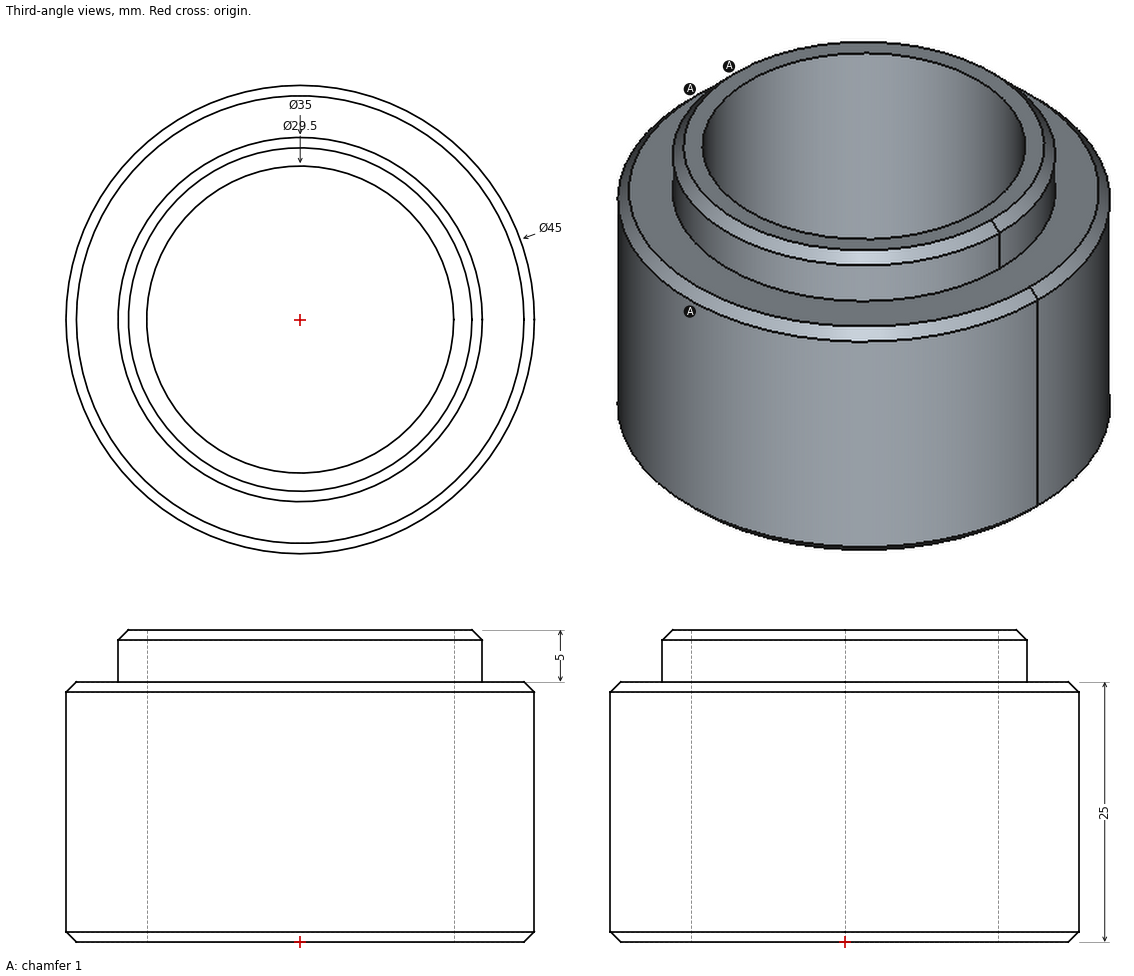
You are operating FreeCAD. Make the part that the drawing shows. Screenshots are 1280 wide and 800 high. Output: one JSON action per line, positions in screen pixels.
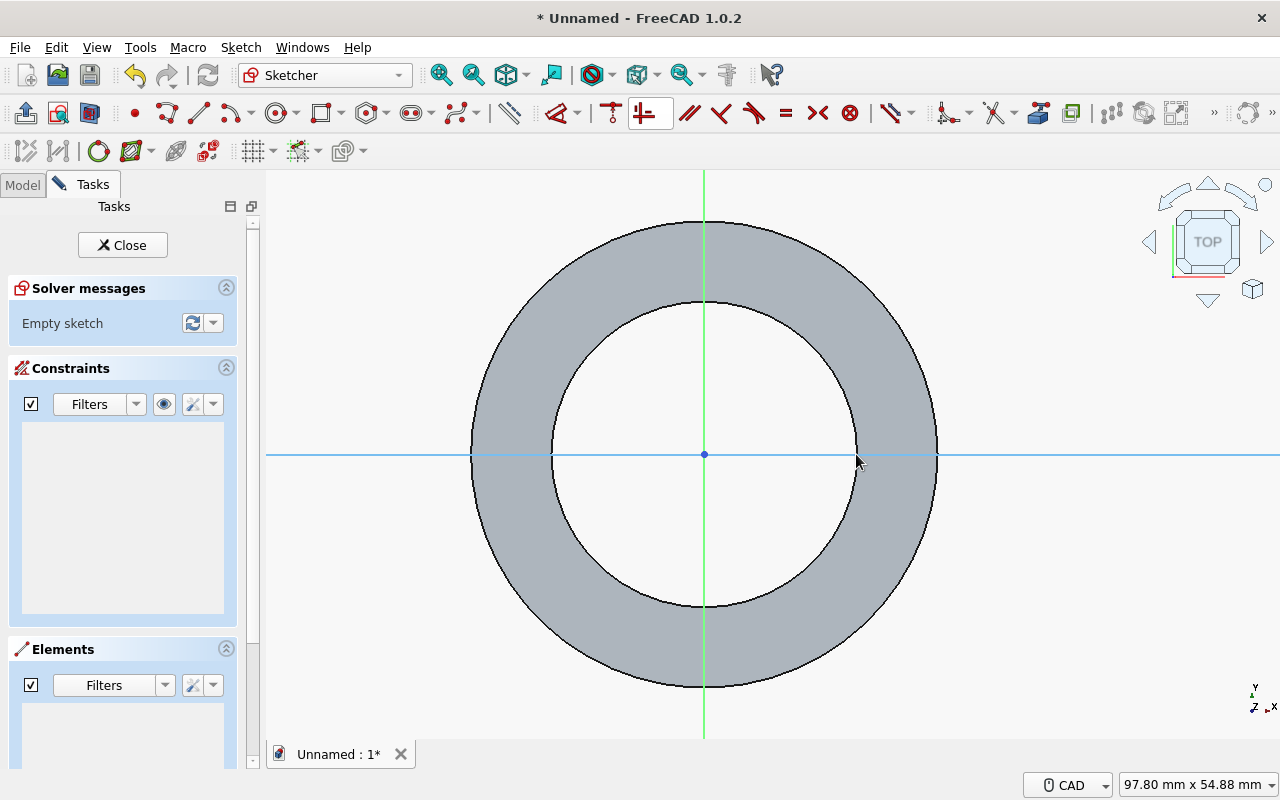
{"action": "key", "text": "g c"}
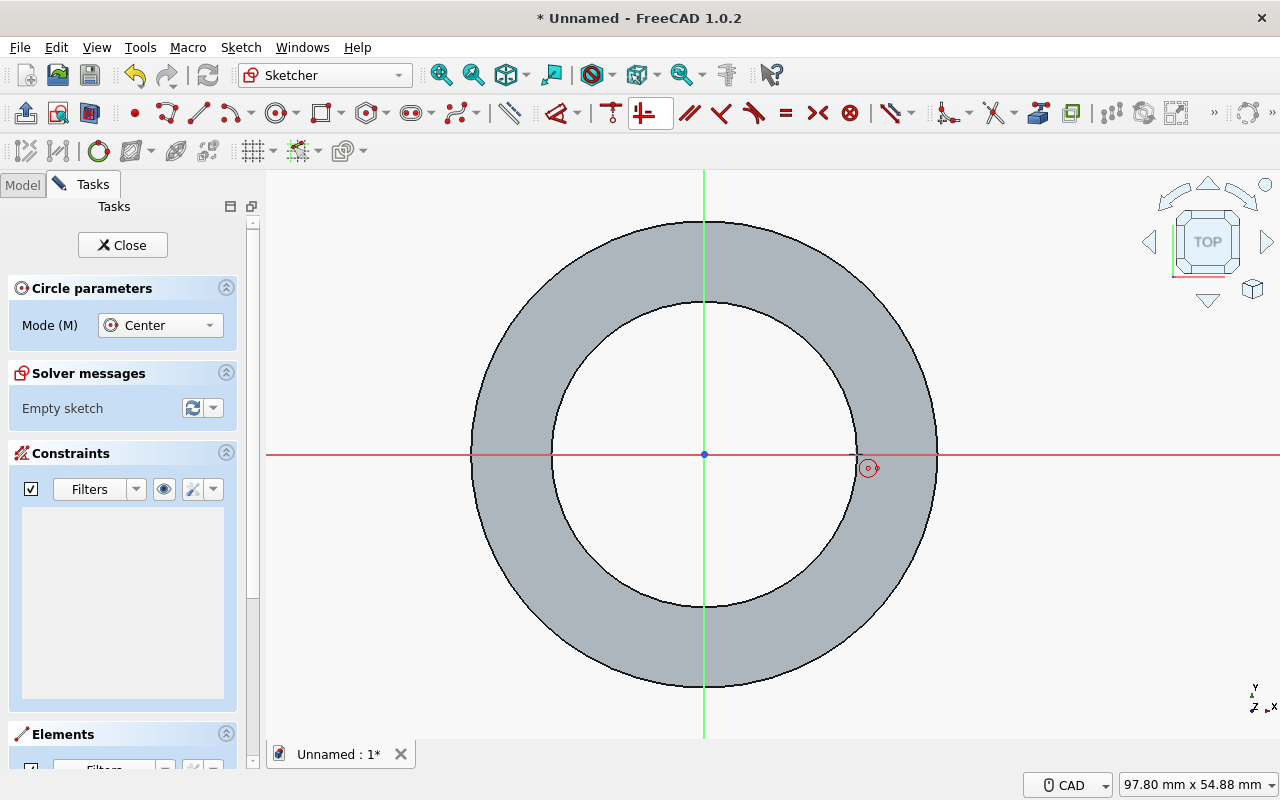
{"action": "left_click", "coordinate": [704, 454]}
{"action": "left_click", "coordinate": [833, 326]}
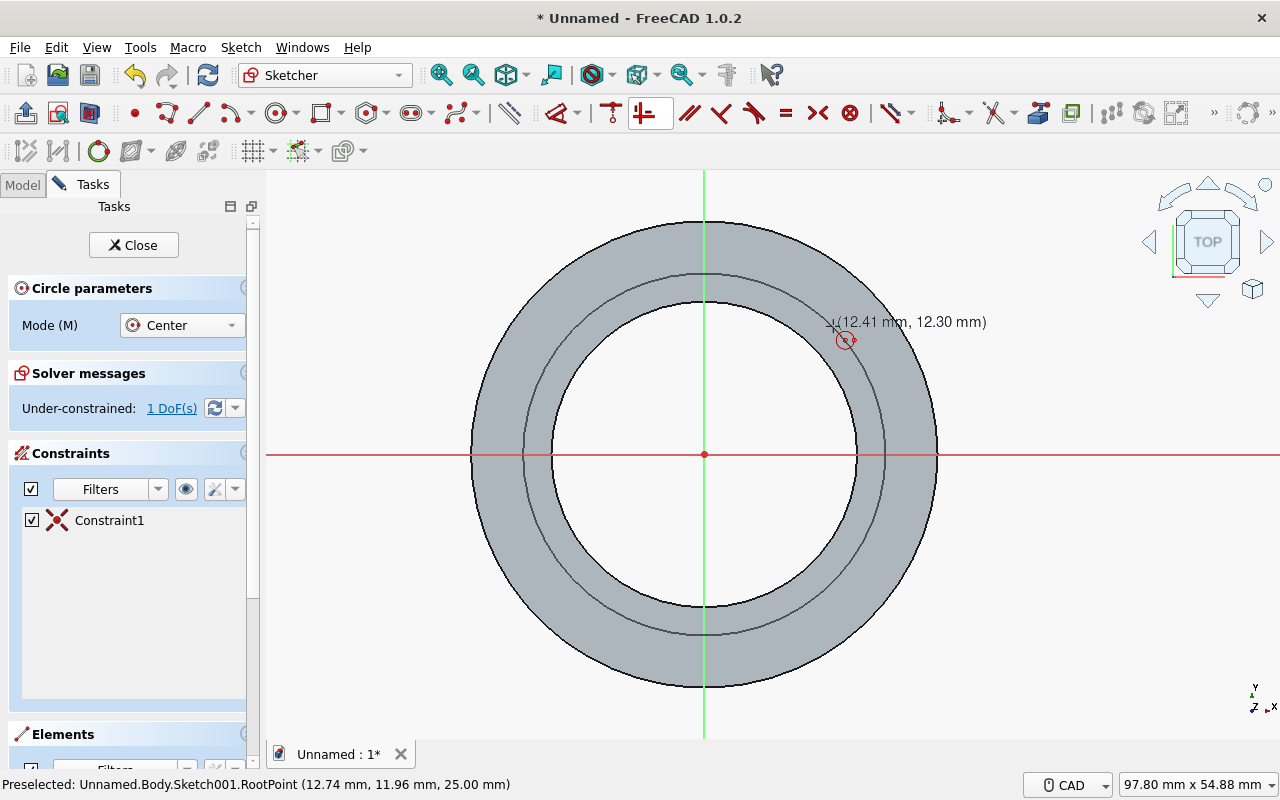
{"action": "left_click", "coordinate": [704, 454]}
{"action": "left_click", "coordinate": [812, 346]}
{"action": "key", "text": "Escape"}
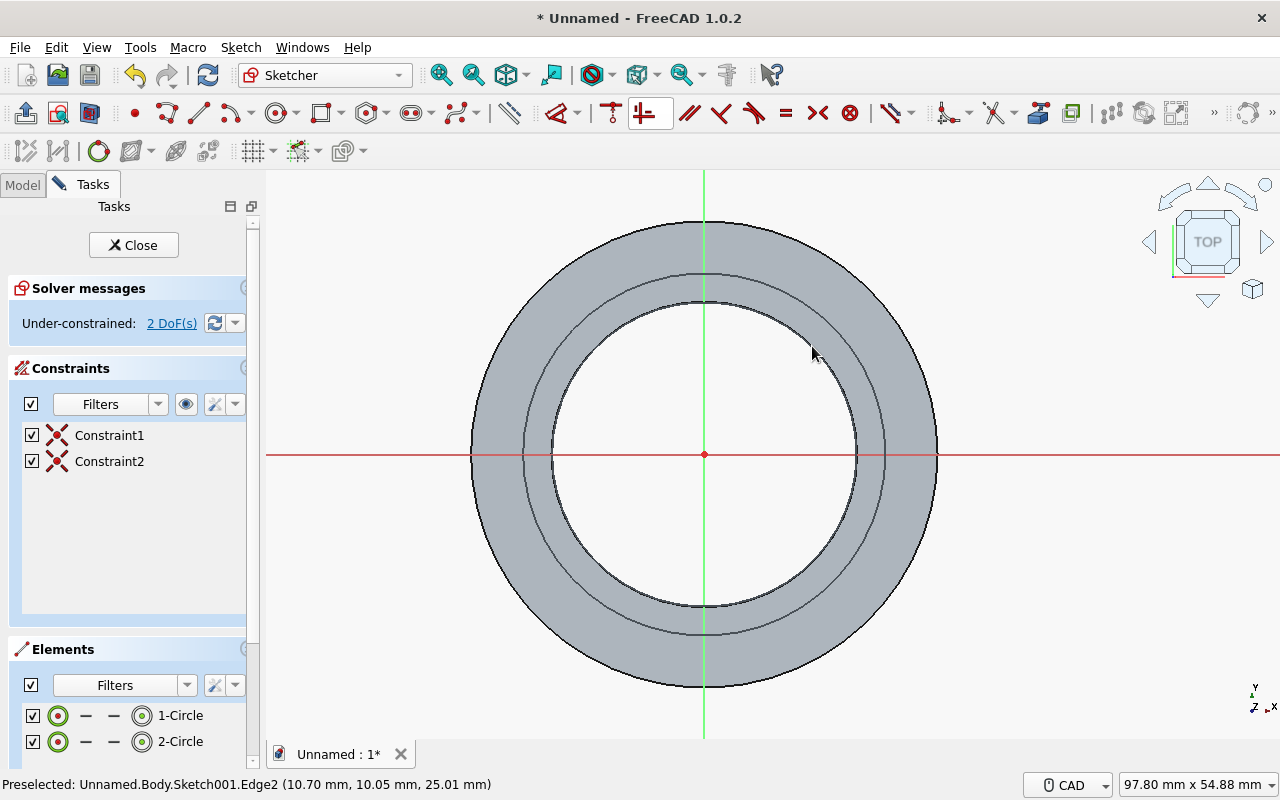
{"action": "left_click", "coordinate": [556, 114]}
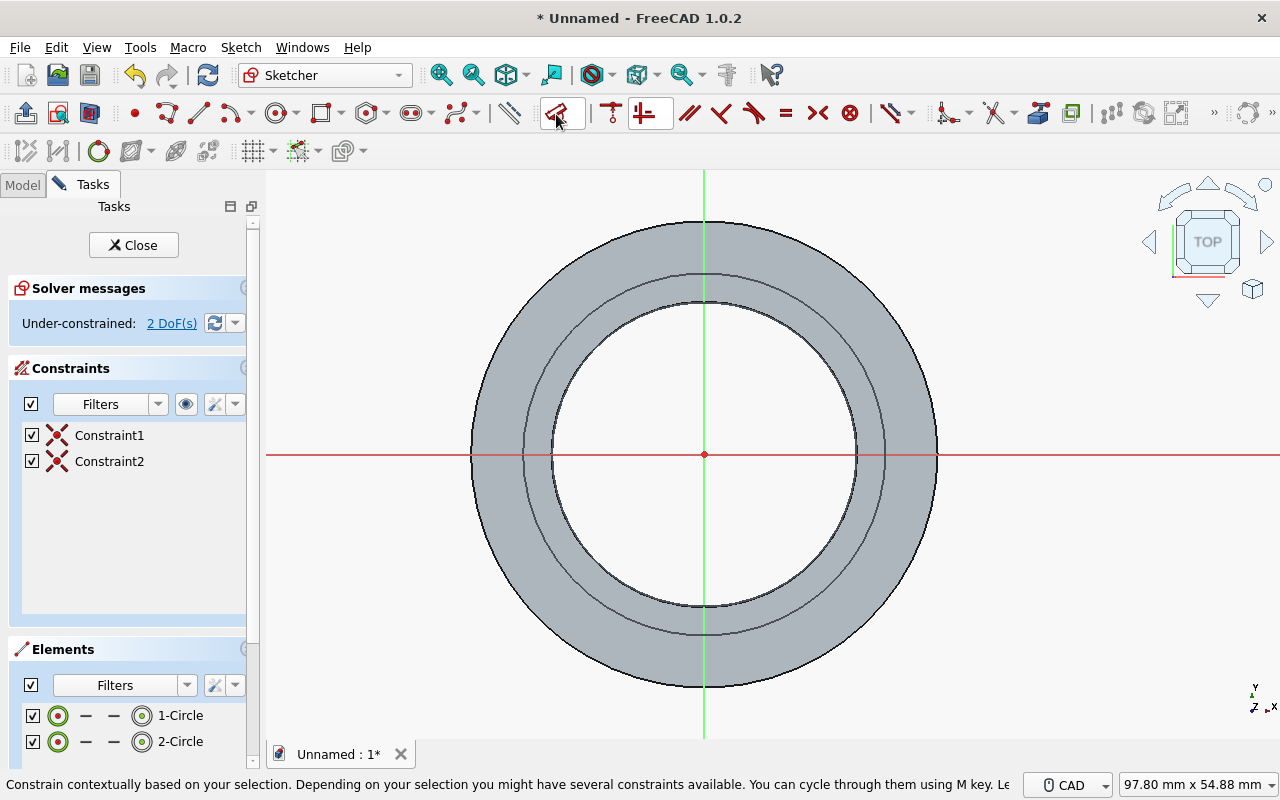
{"action": "left_click", "coordinate": [832, 326]}
{"action": "left_click", "coordinate": [855, 303]}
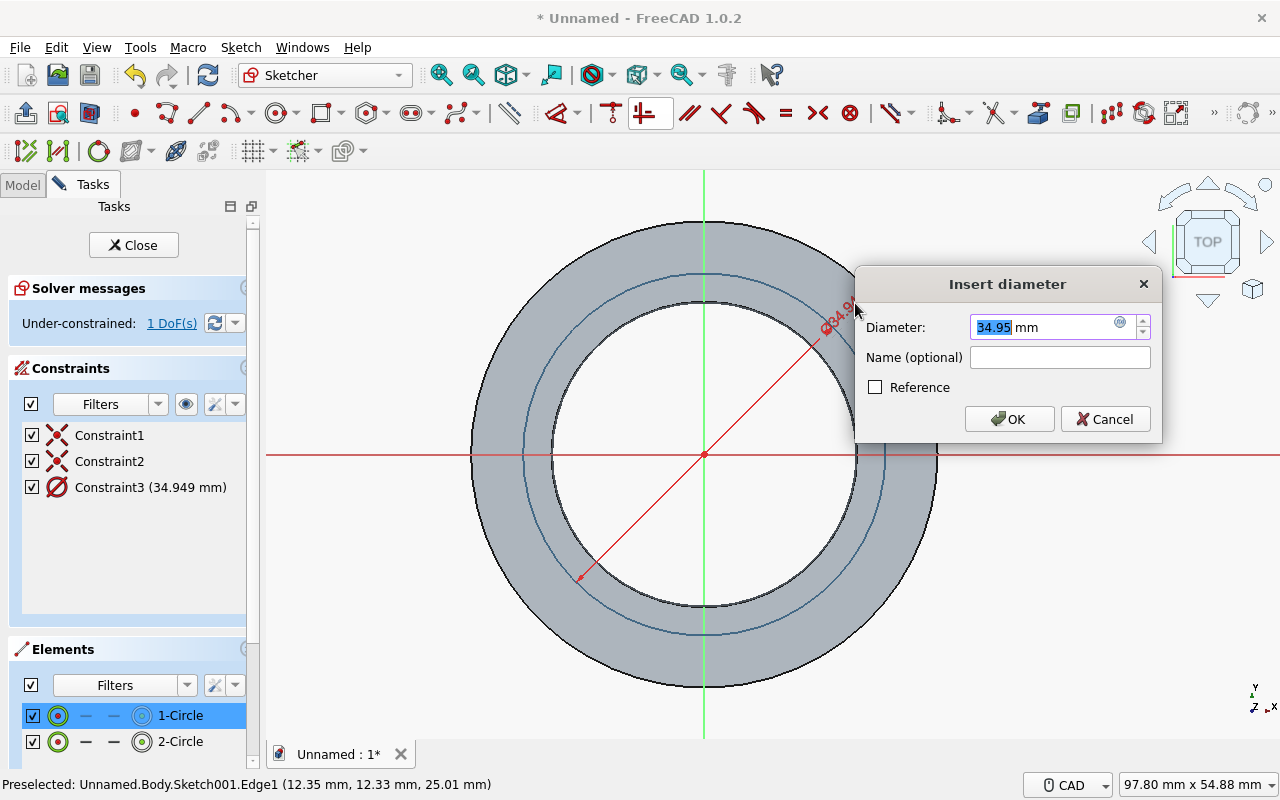
{"action": "type", "text": "35"}
{"action": "key", "text": "Return"}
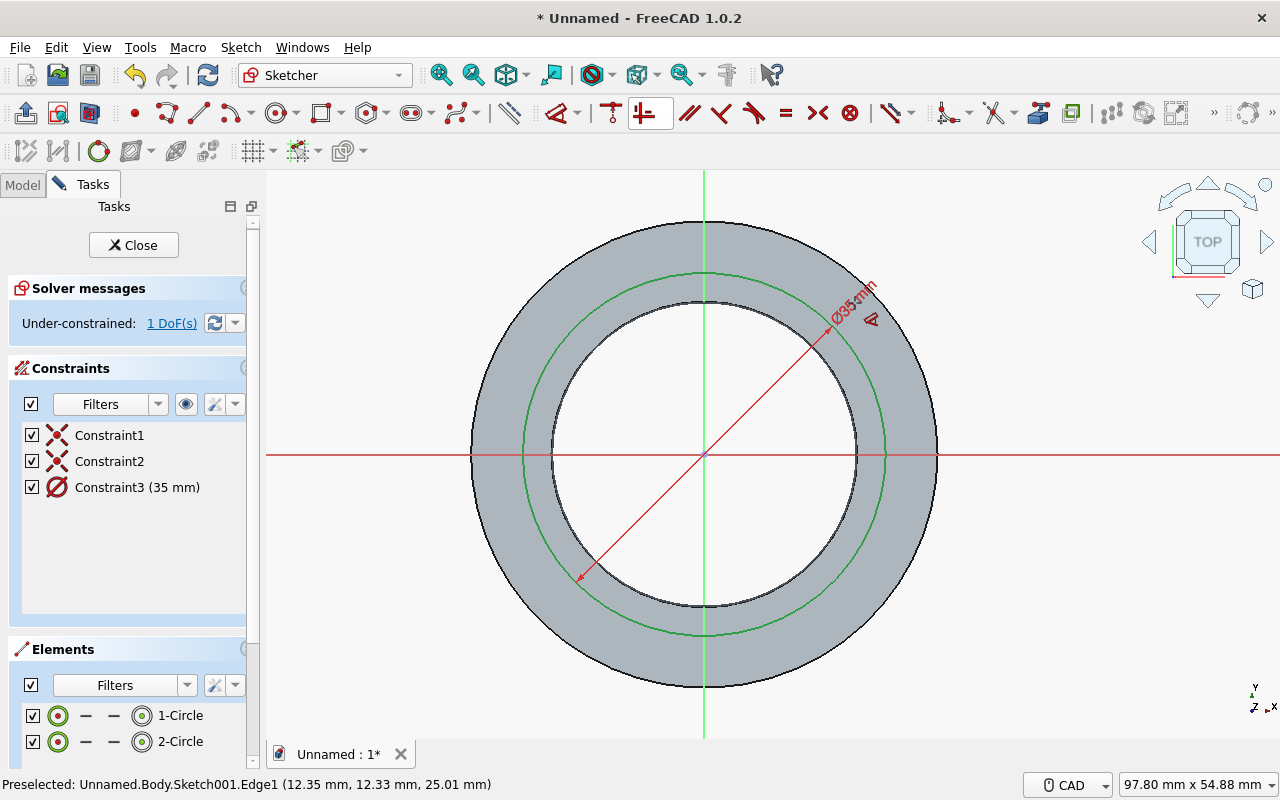
{"action": "left_click", "coordinate": [812, 347]}
{"action": "left_click", "coordinate": [903, 396]}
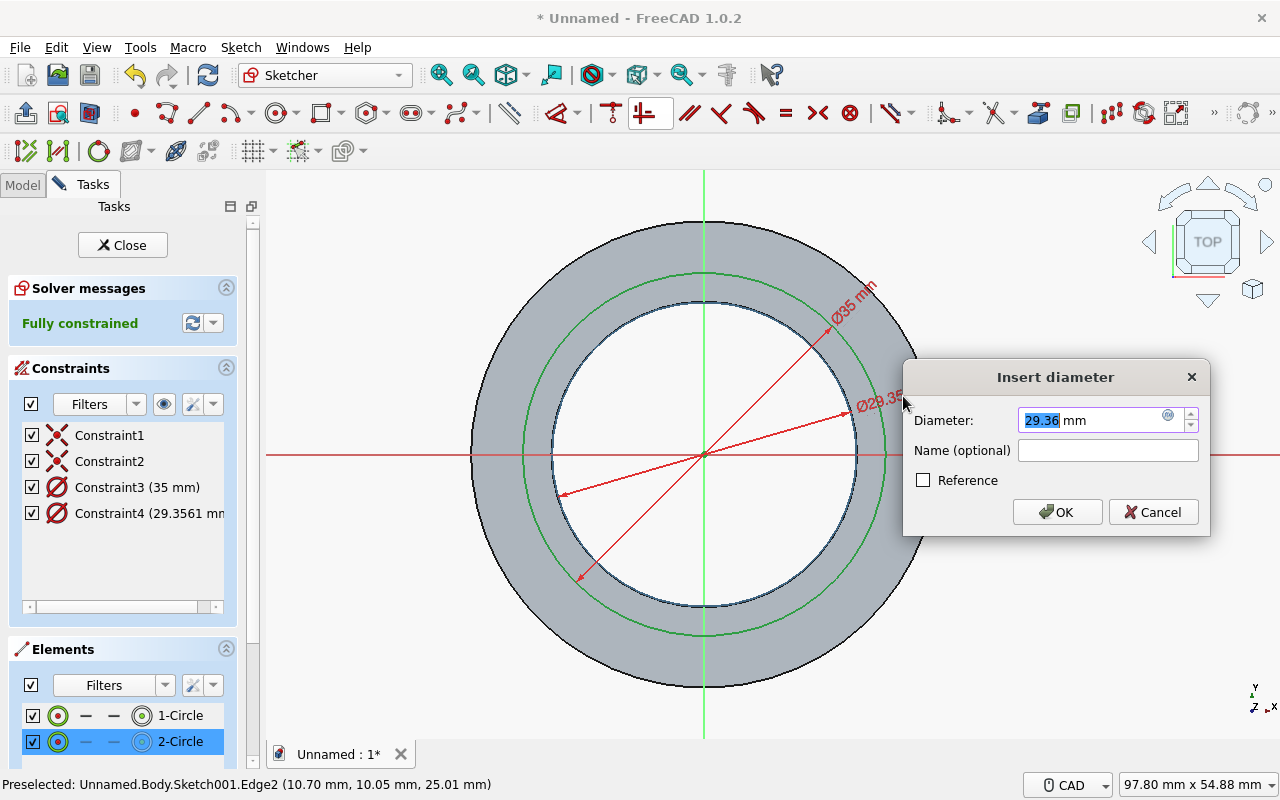
{"action": "type", "text": "29.5"}
{"action": "key", "text": "Return"}
{"action": "key", "text": "Escape"}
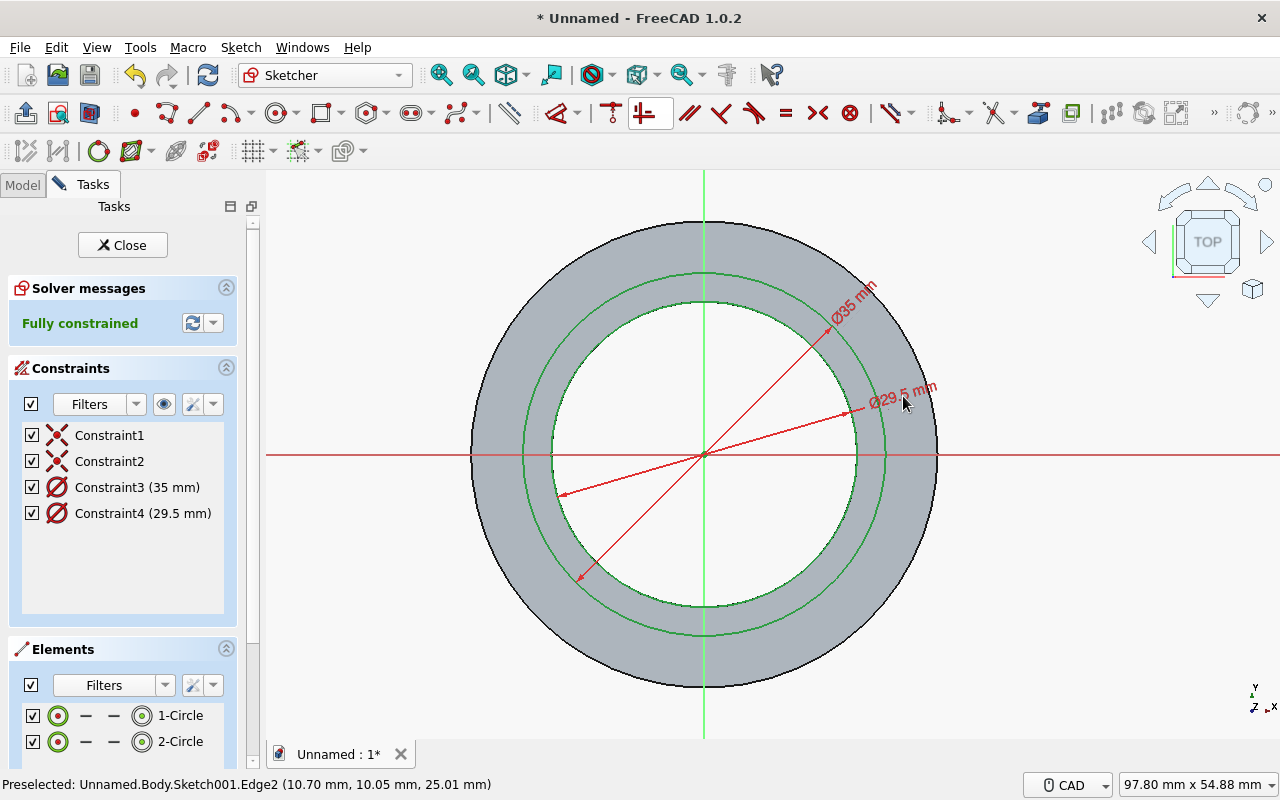
{"action": "left_click", "coordinate": [123, 245]}